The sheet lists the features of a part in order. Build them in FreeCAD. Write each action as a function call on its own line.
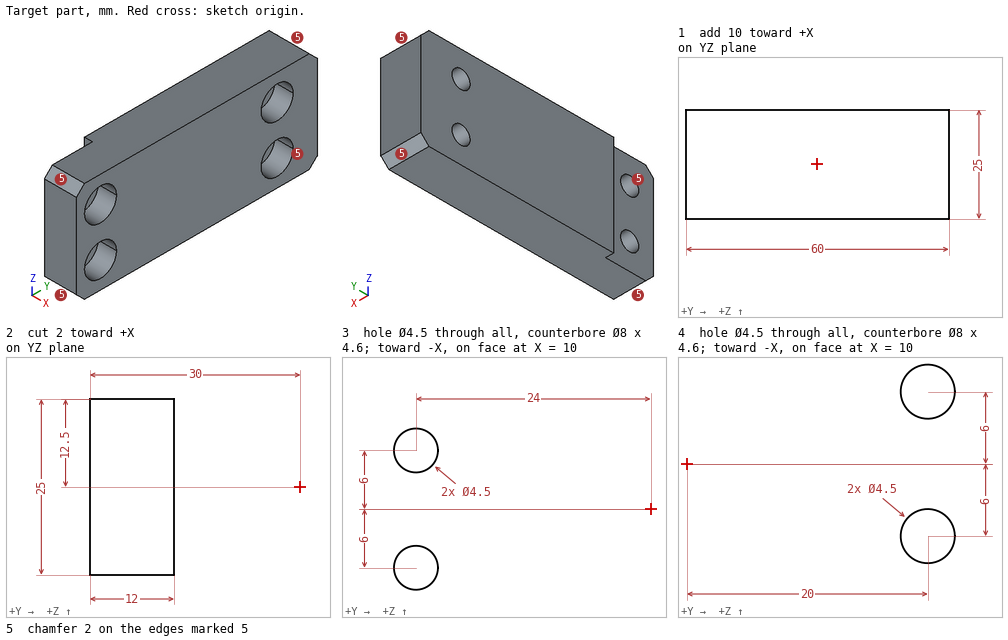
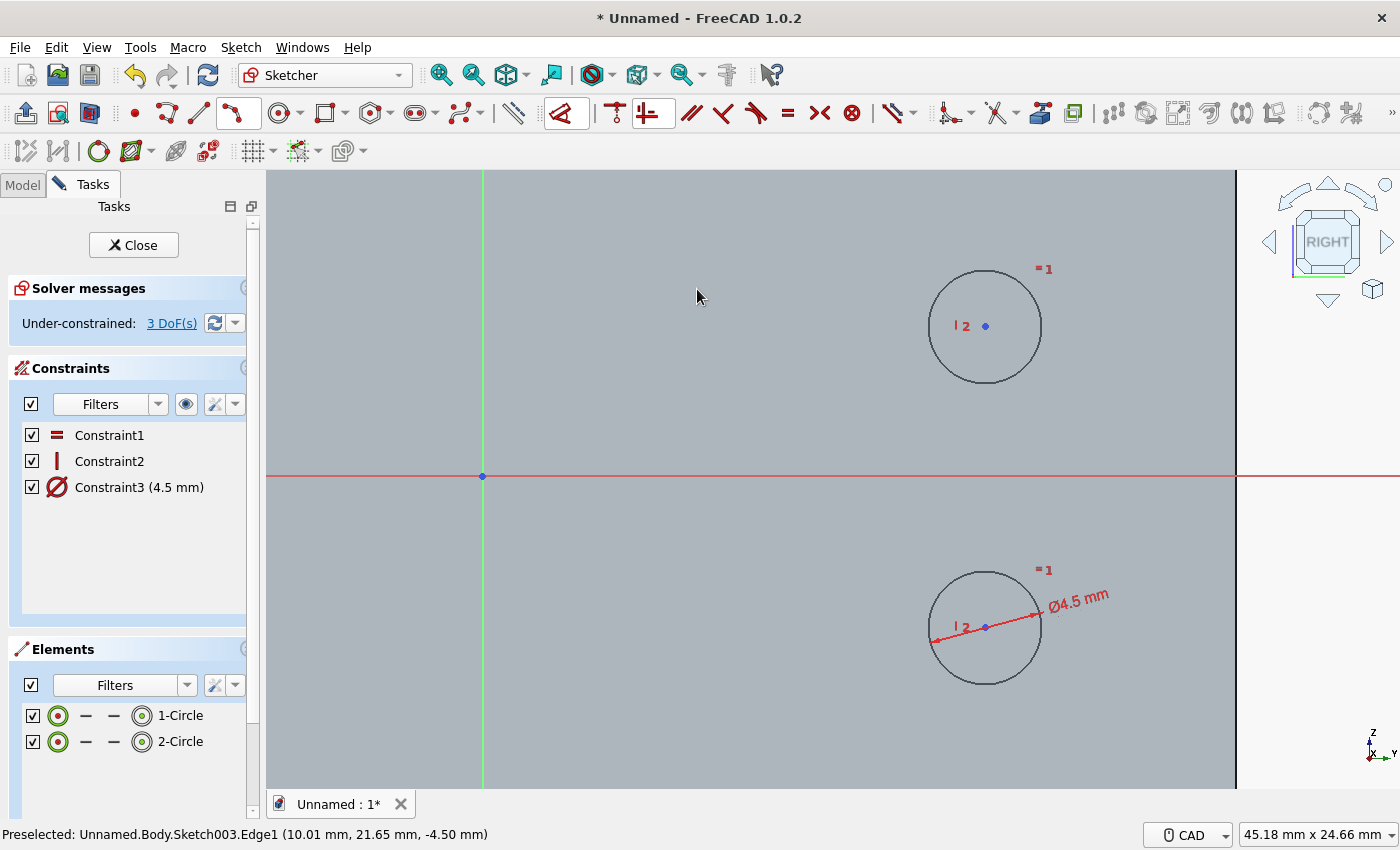
click(985, 628)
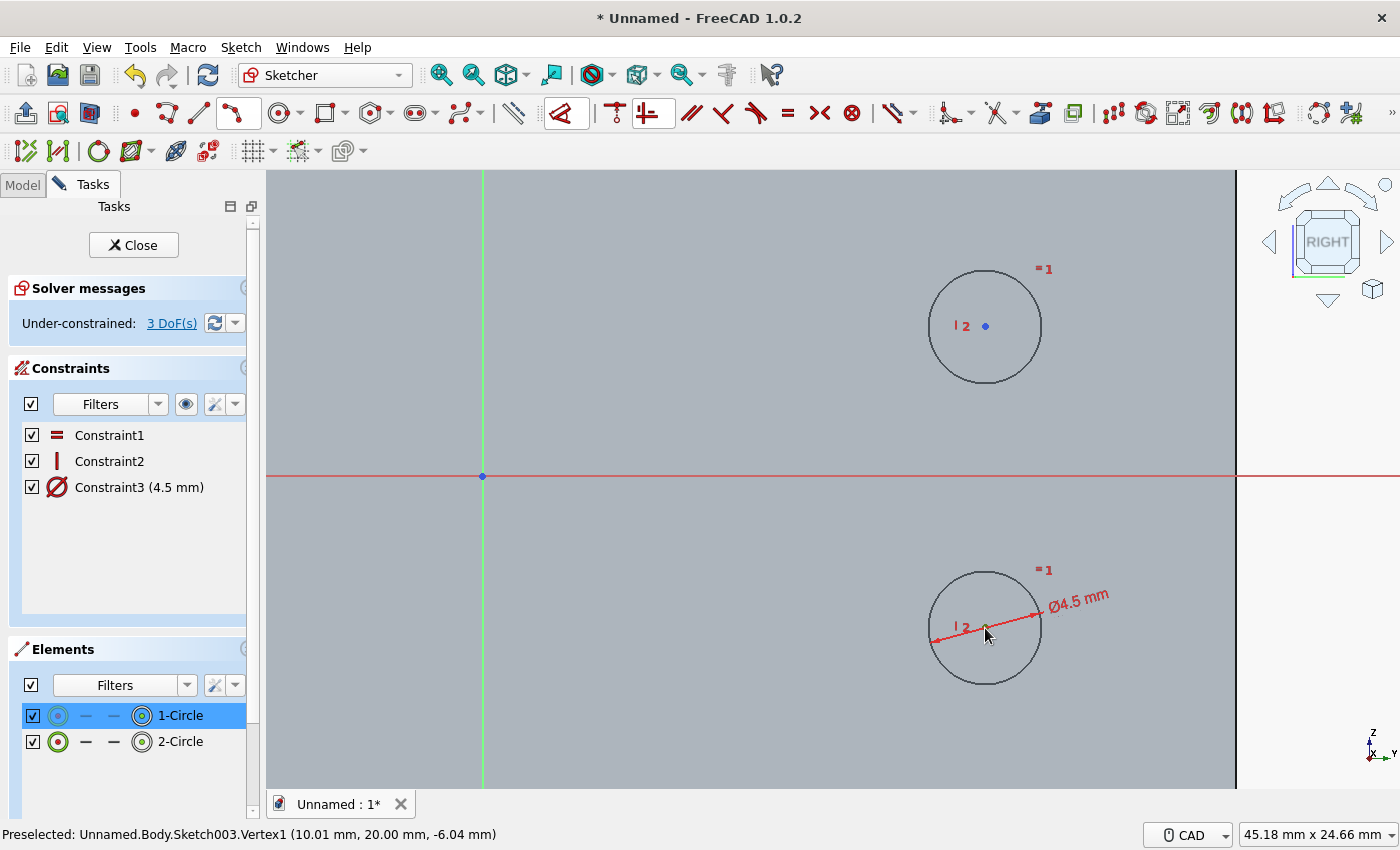
key(i)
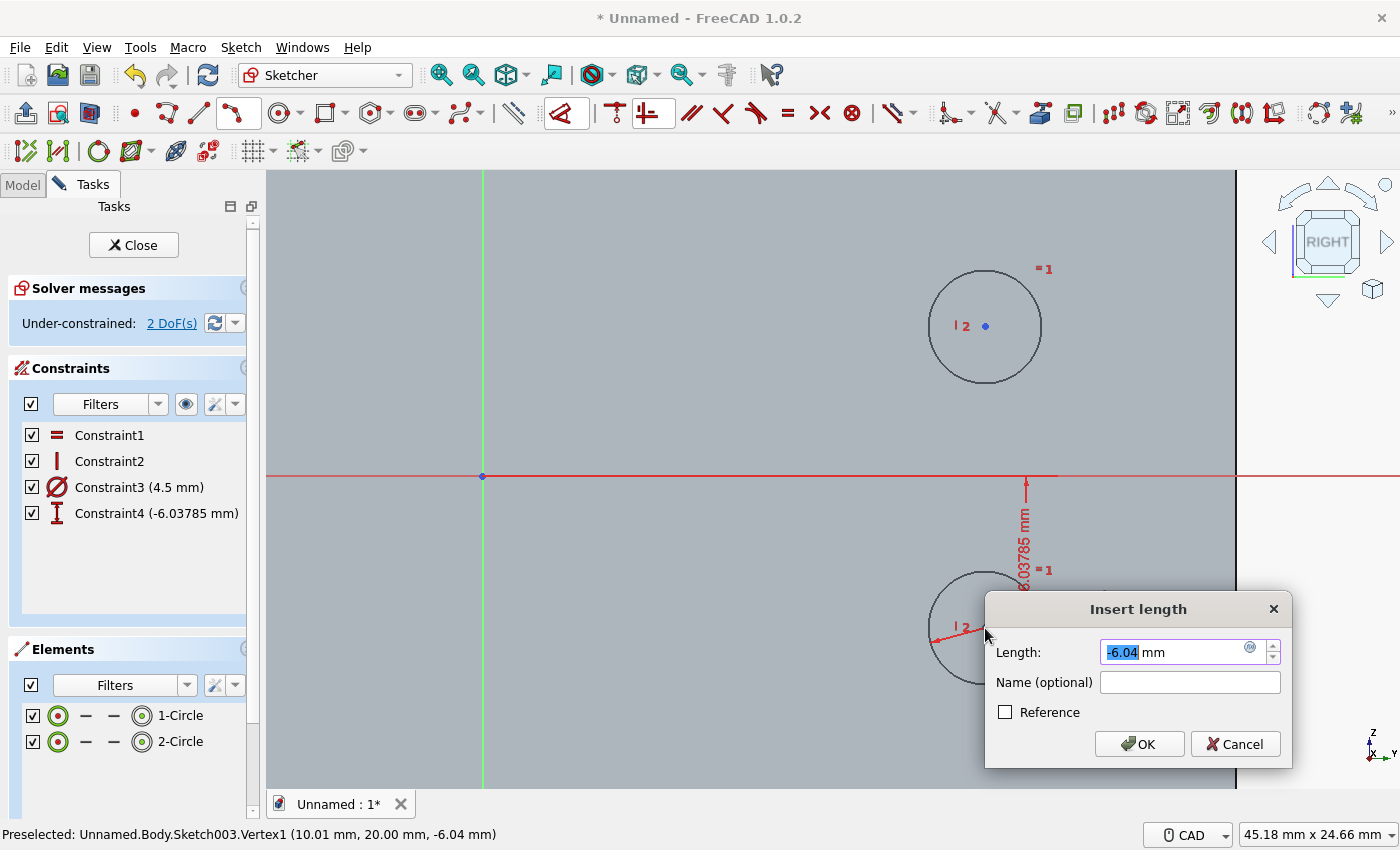
text(-6)
key(Return)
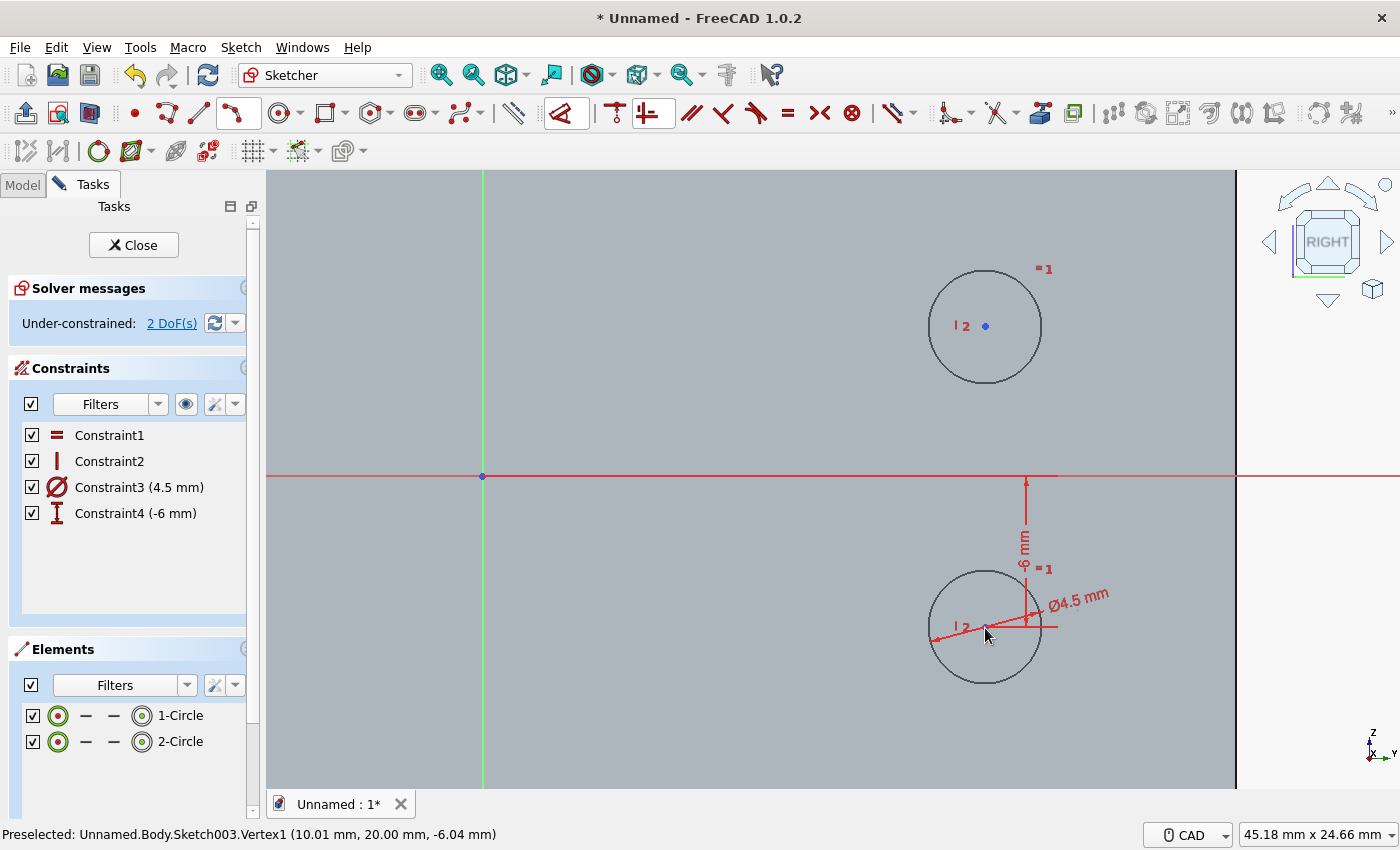
click(985, 327)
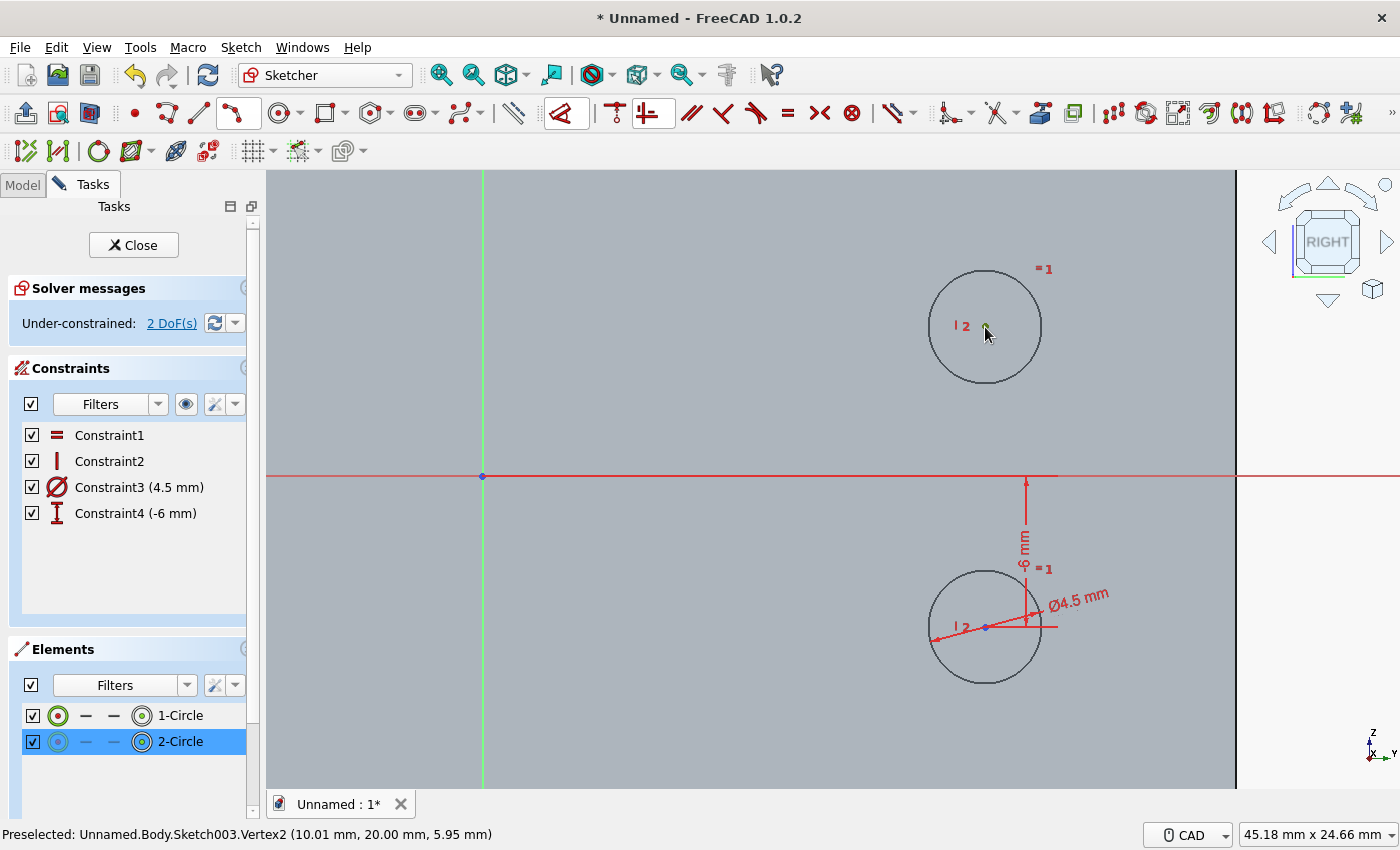
key(i)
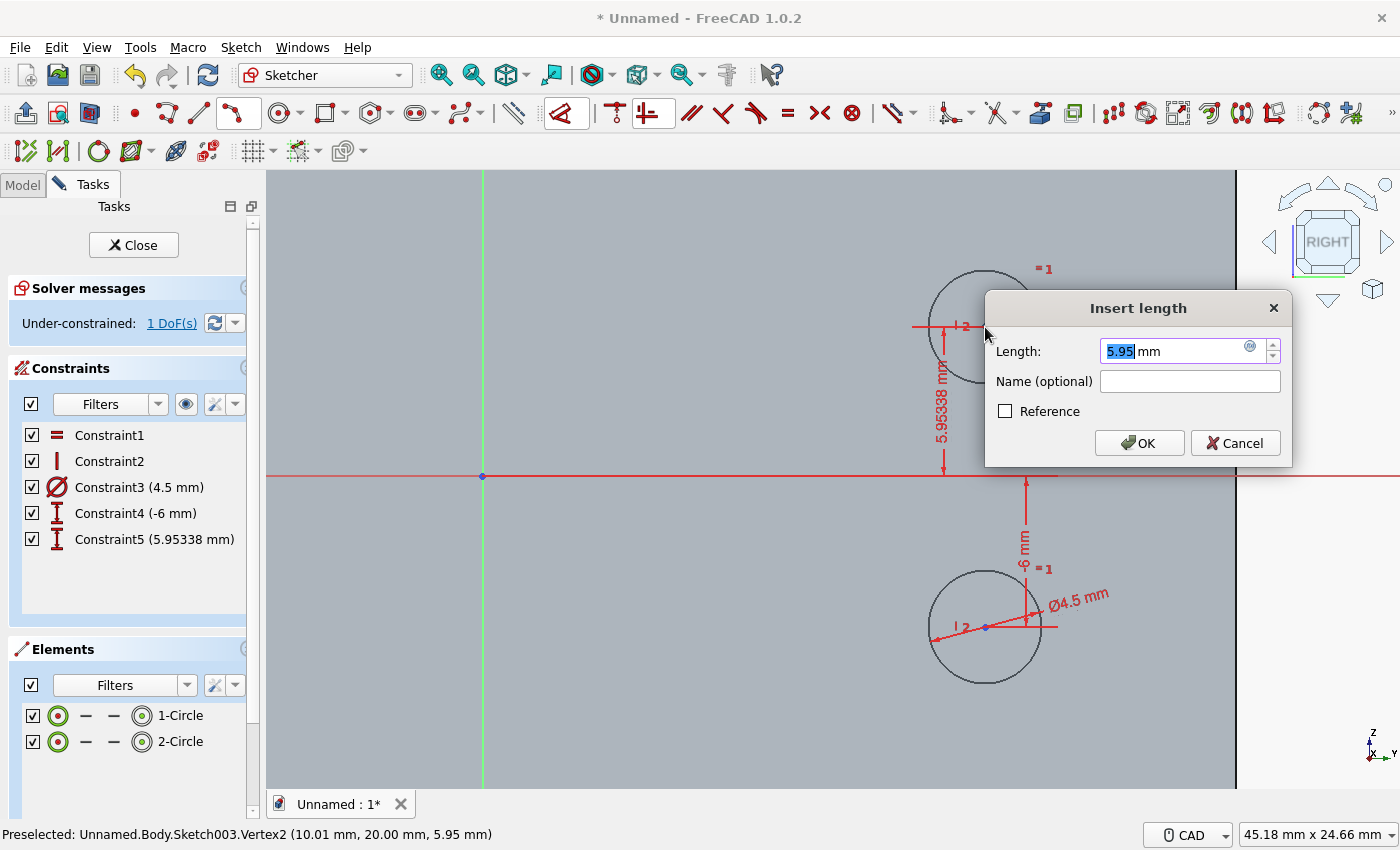
text(6)
key(Return)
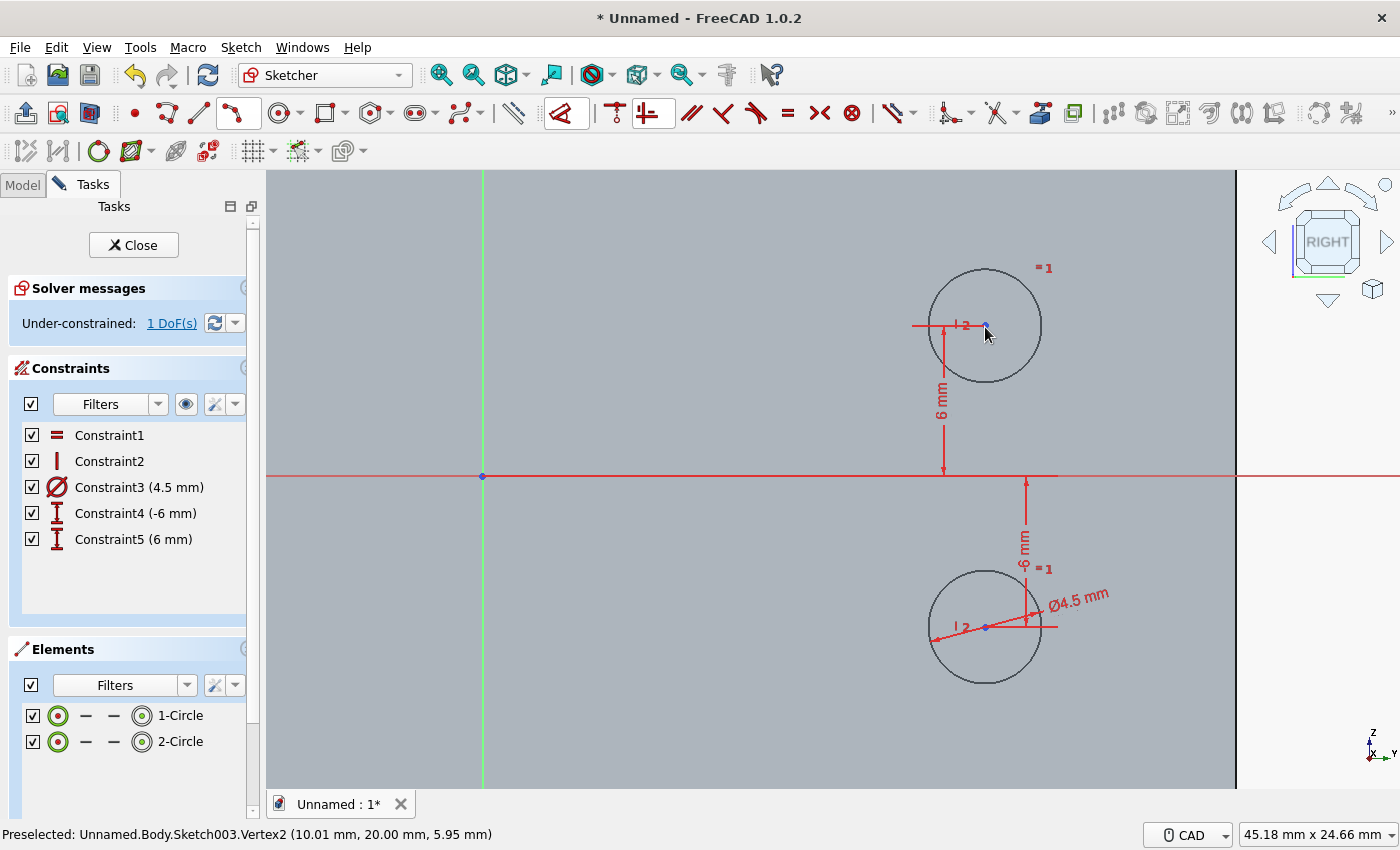
click(985, 627)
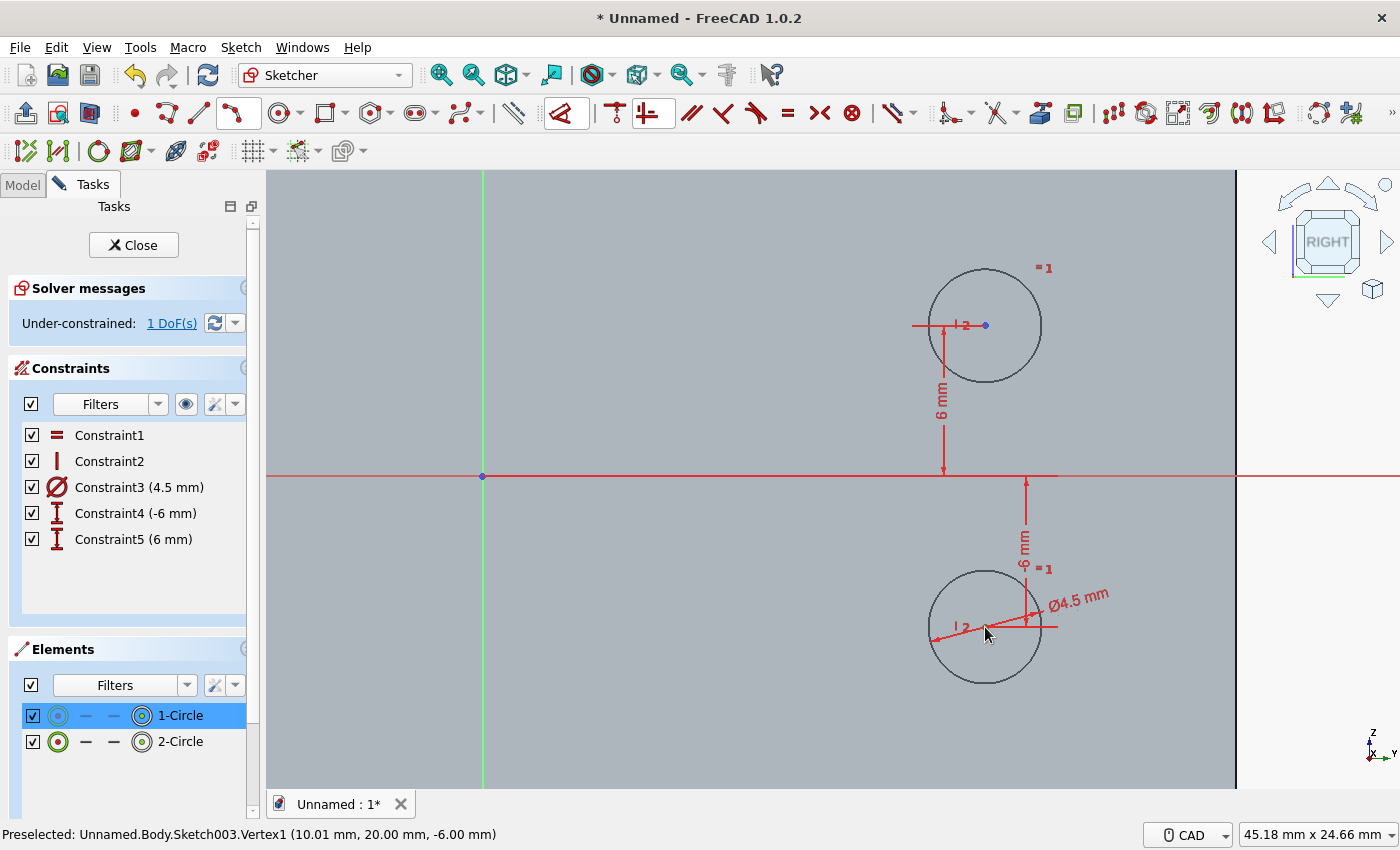
click(584, 114)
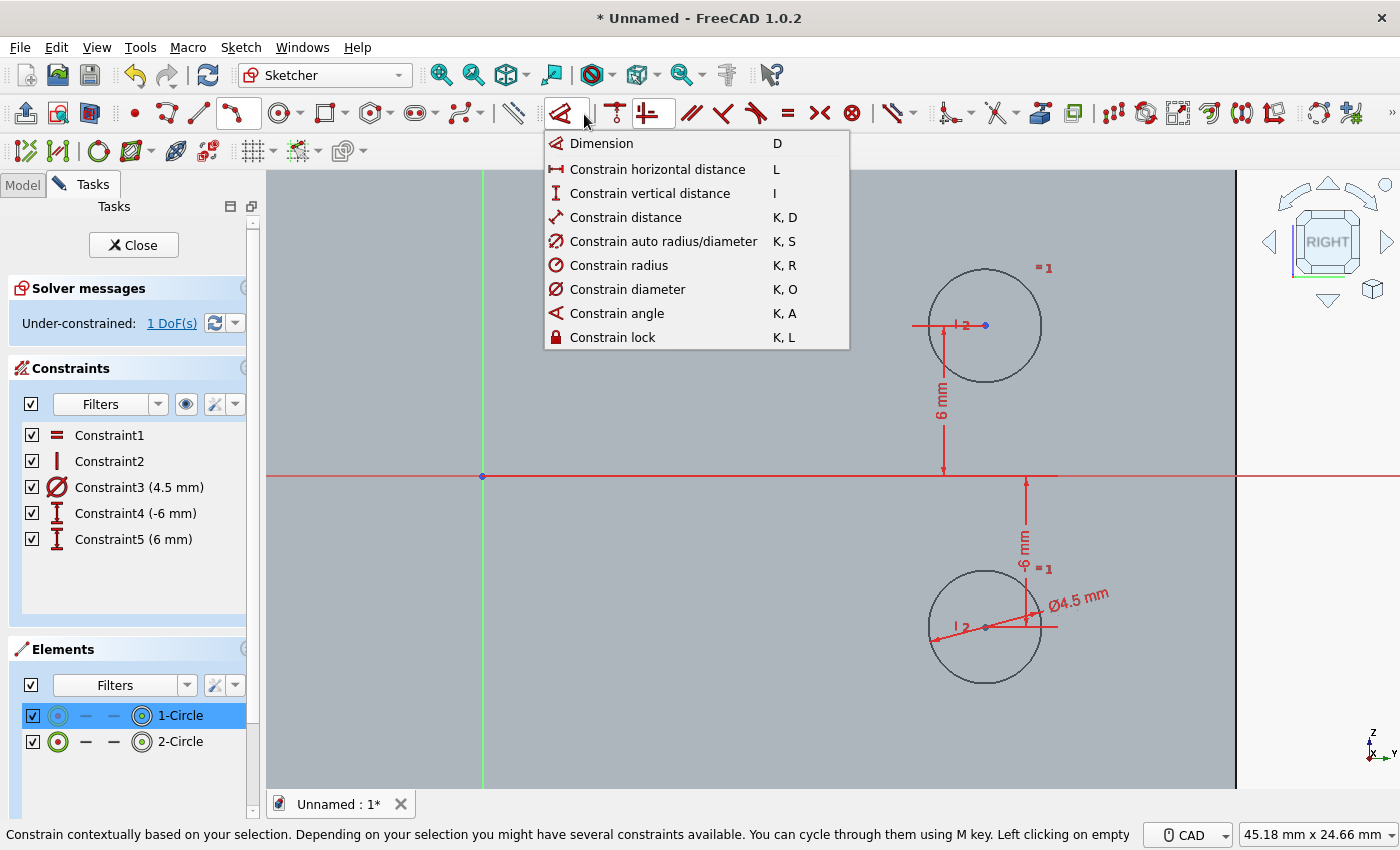
click(697, 169)